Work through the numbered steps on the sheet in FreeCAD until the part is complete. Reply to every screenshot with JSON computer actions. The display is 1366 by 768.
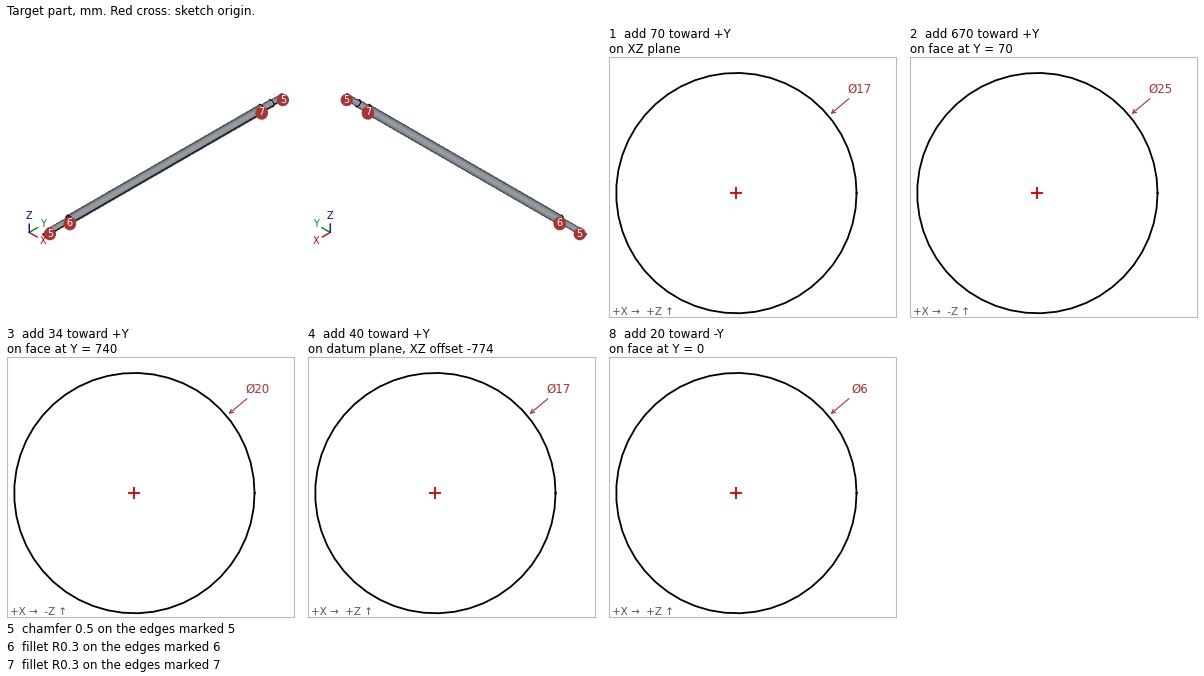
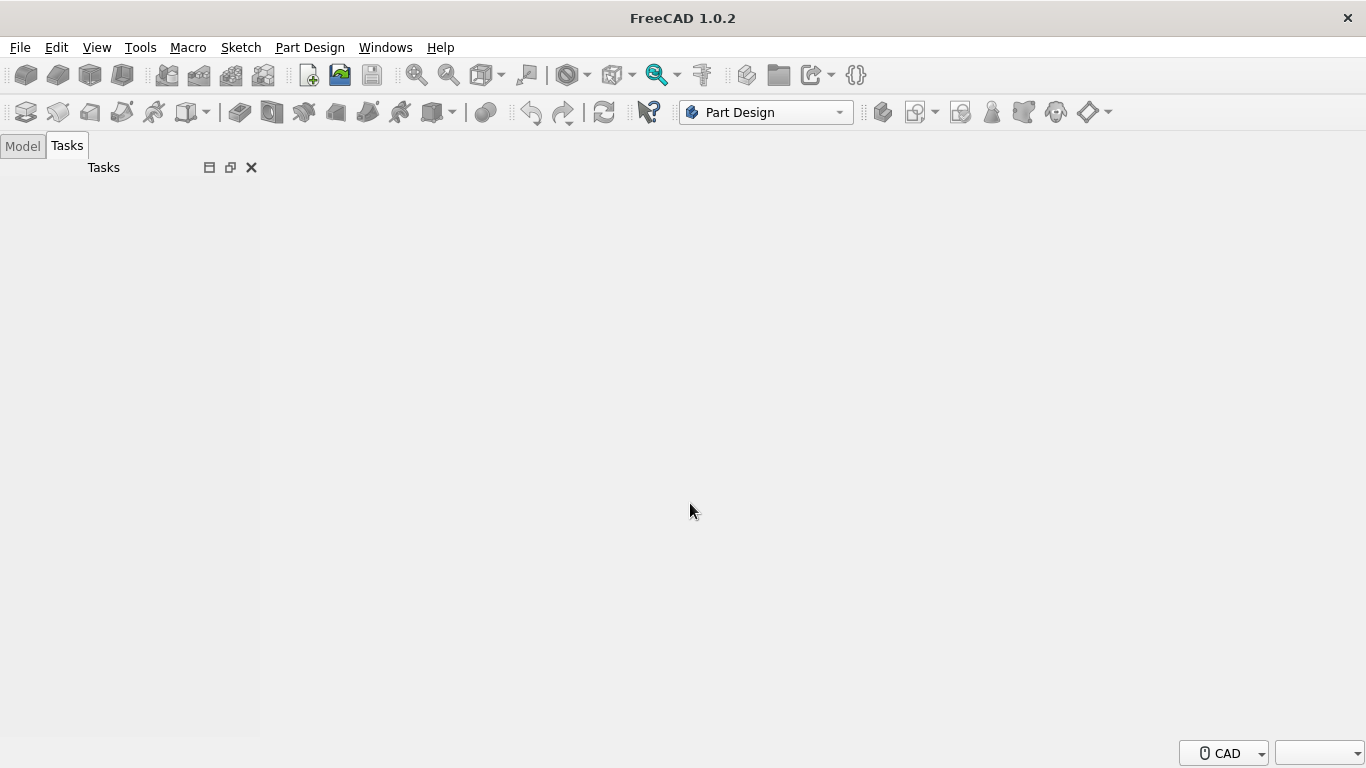
{"action": "left_click", "coordinate": [308, 76]}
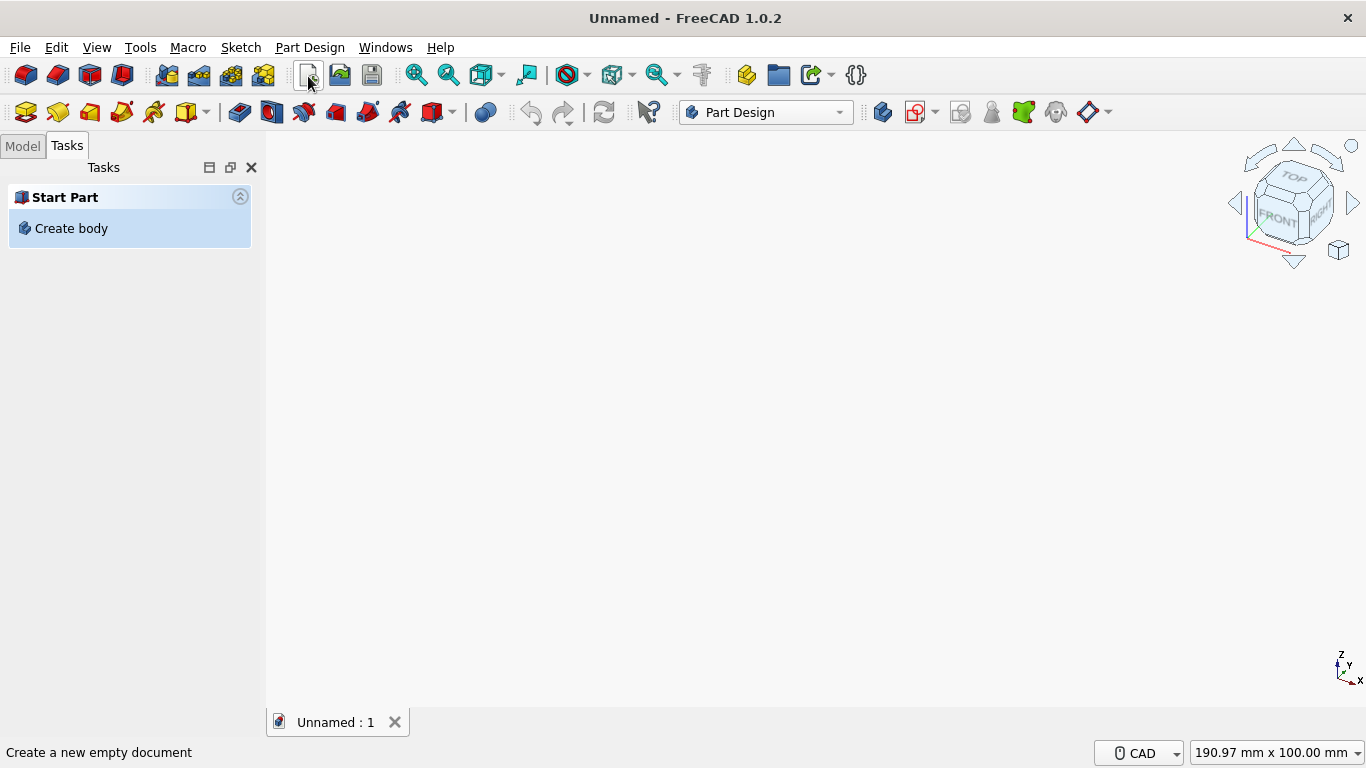
{"action": "left_click", "coordinate": [916, 112]}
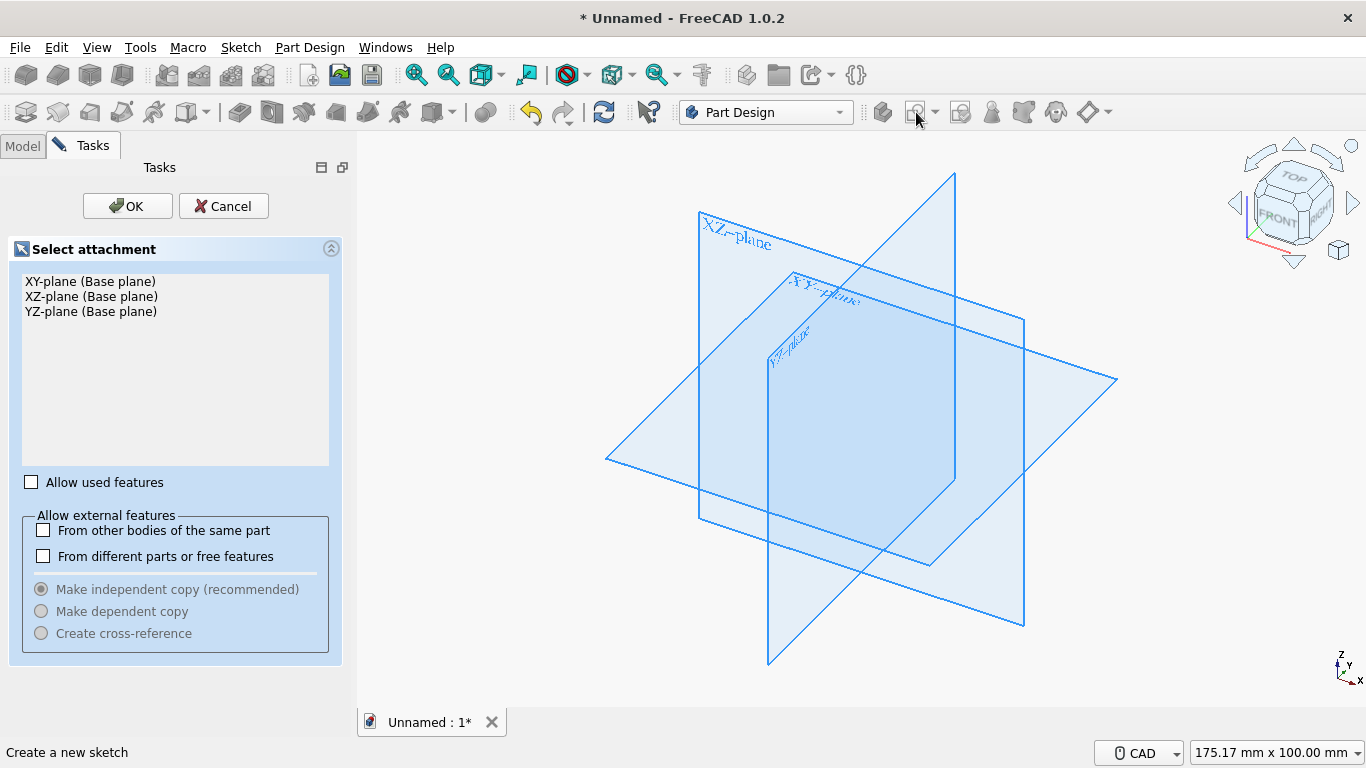
{"action": "left_click", "coordinate": [82, 296]}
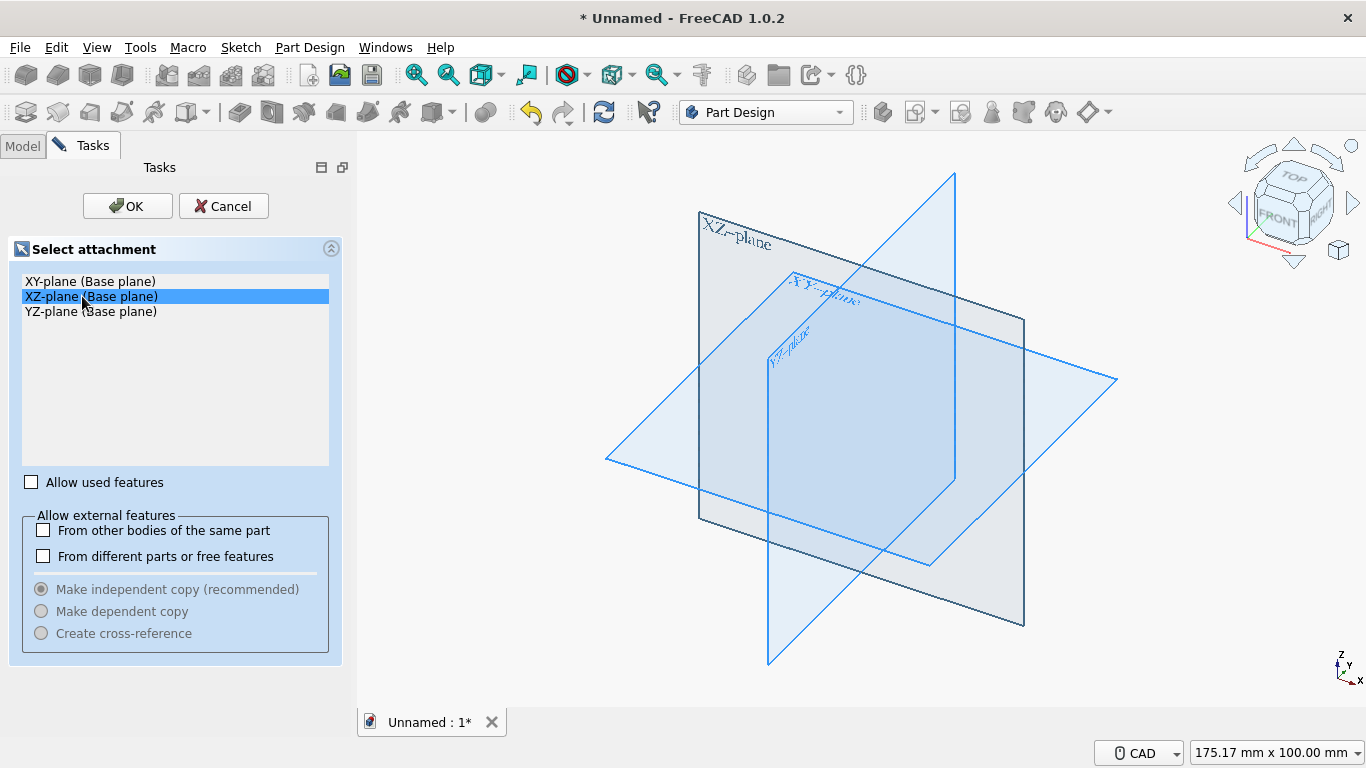
{"action": "left_click", "coordinate": [128, 206]}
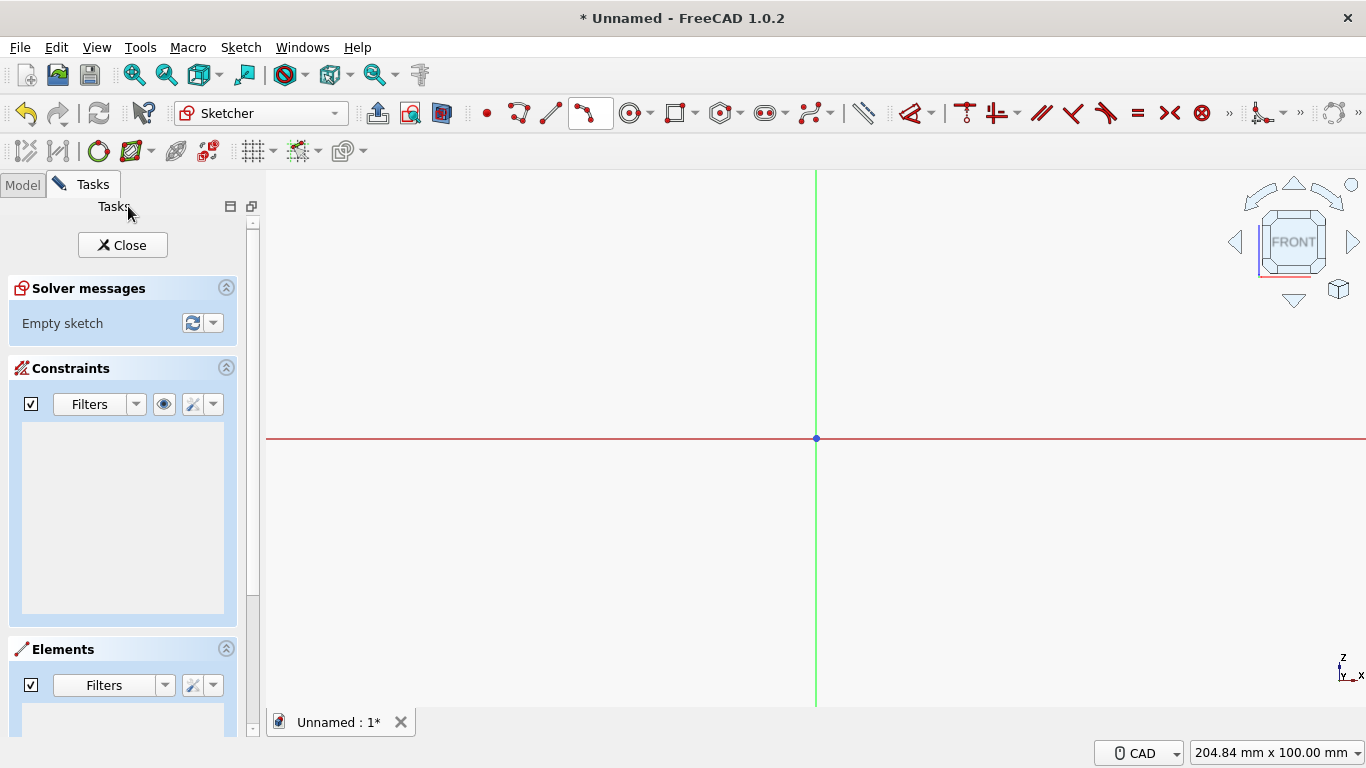
{"action": "scroll", "coordinate": [838, 438], "scroll_direction": "up", "scroll_amount": 7}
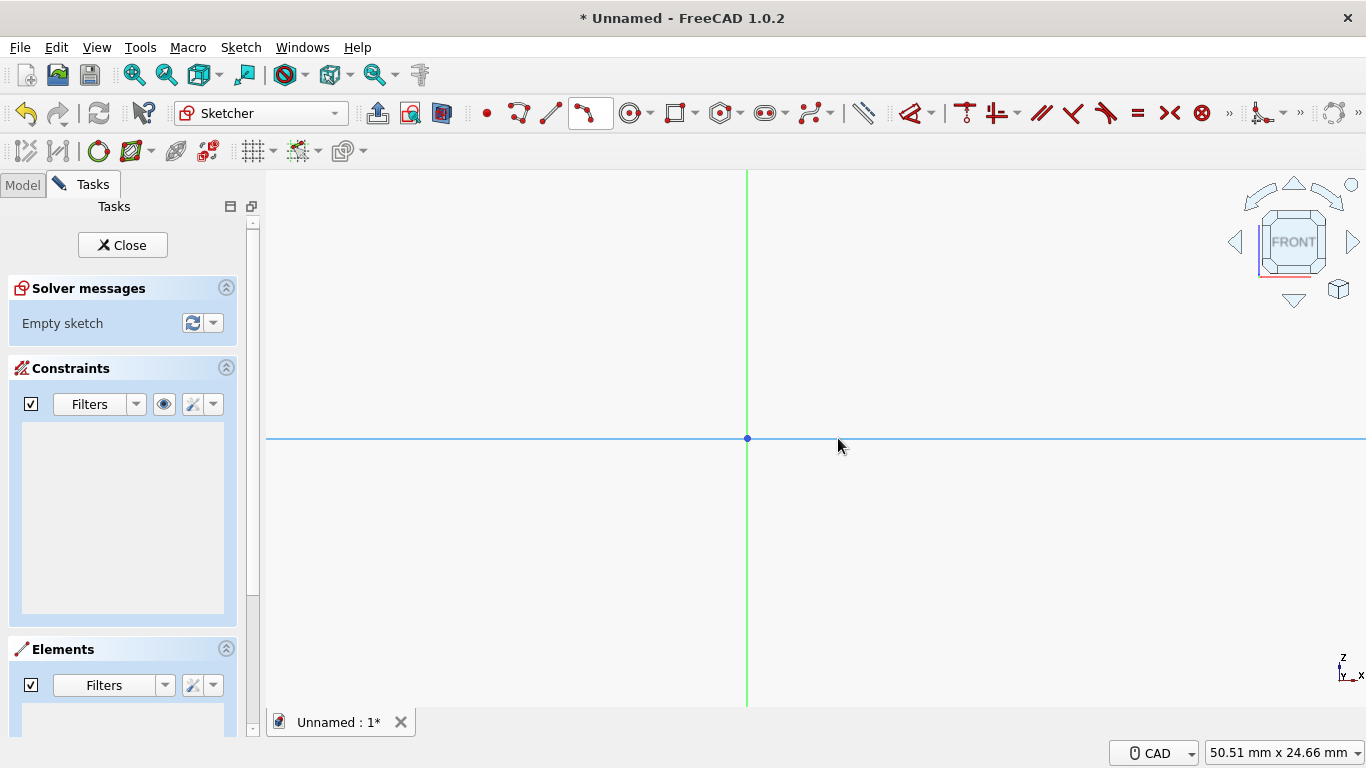
{"action": "left_click", "coordinate": [630, 114]}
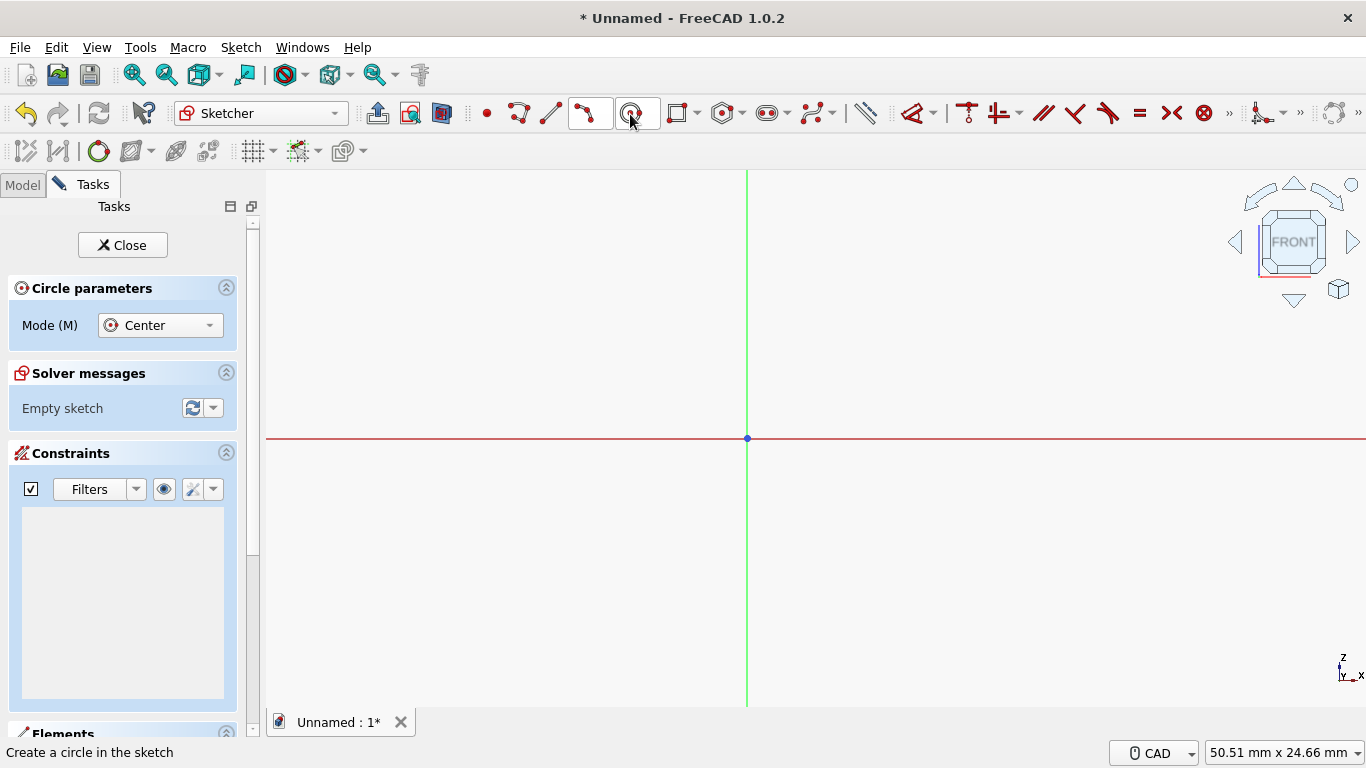
{"action": "left_click", "coordinate": [747, 438]}
{"action": "left_click", "coordinate": [878, 308]}
{"action": "key", "text": "Escape"}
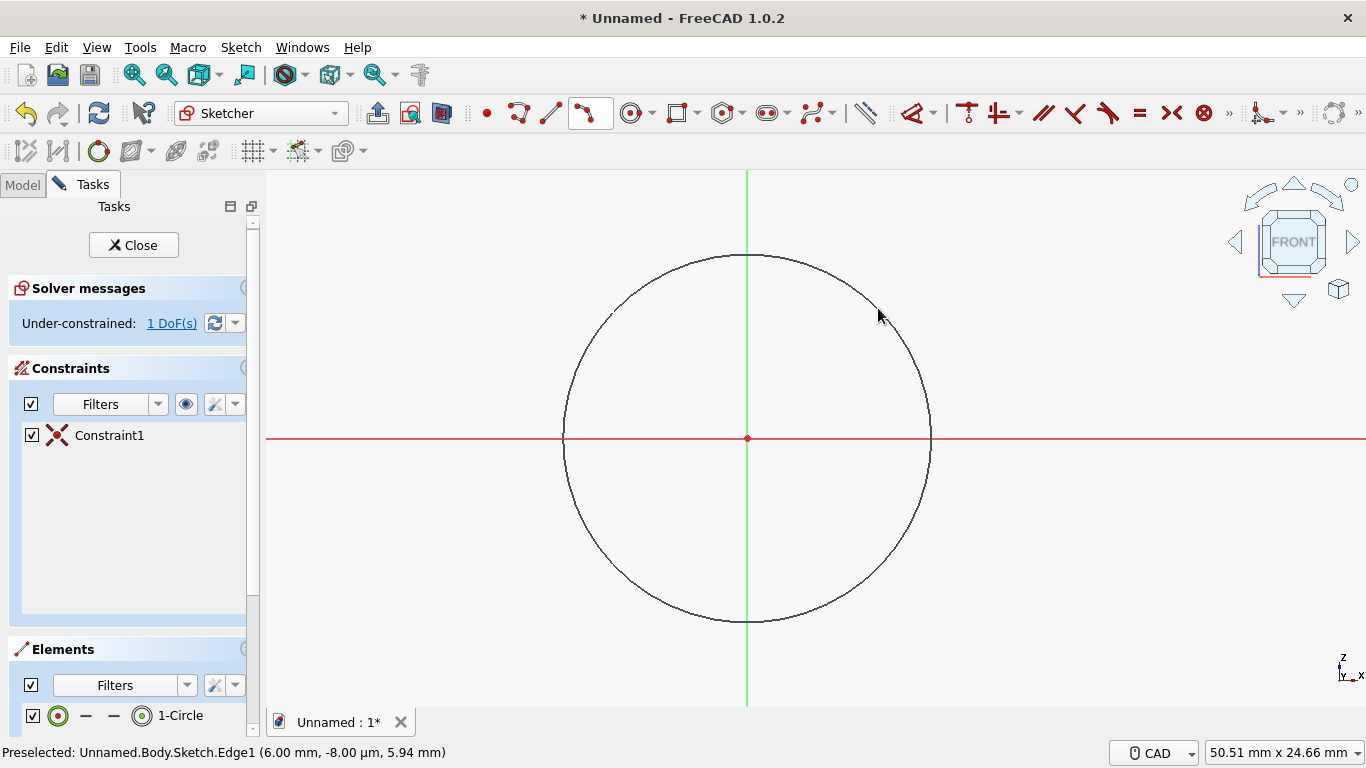
{"action": "left_click", "coordinate": [912, 114]}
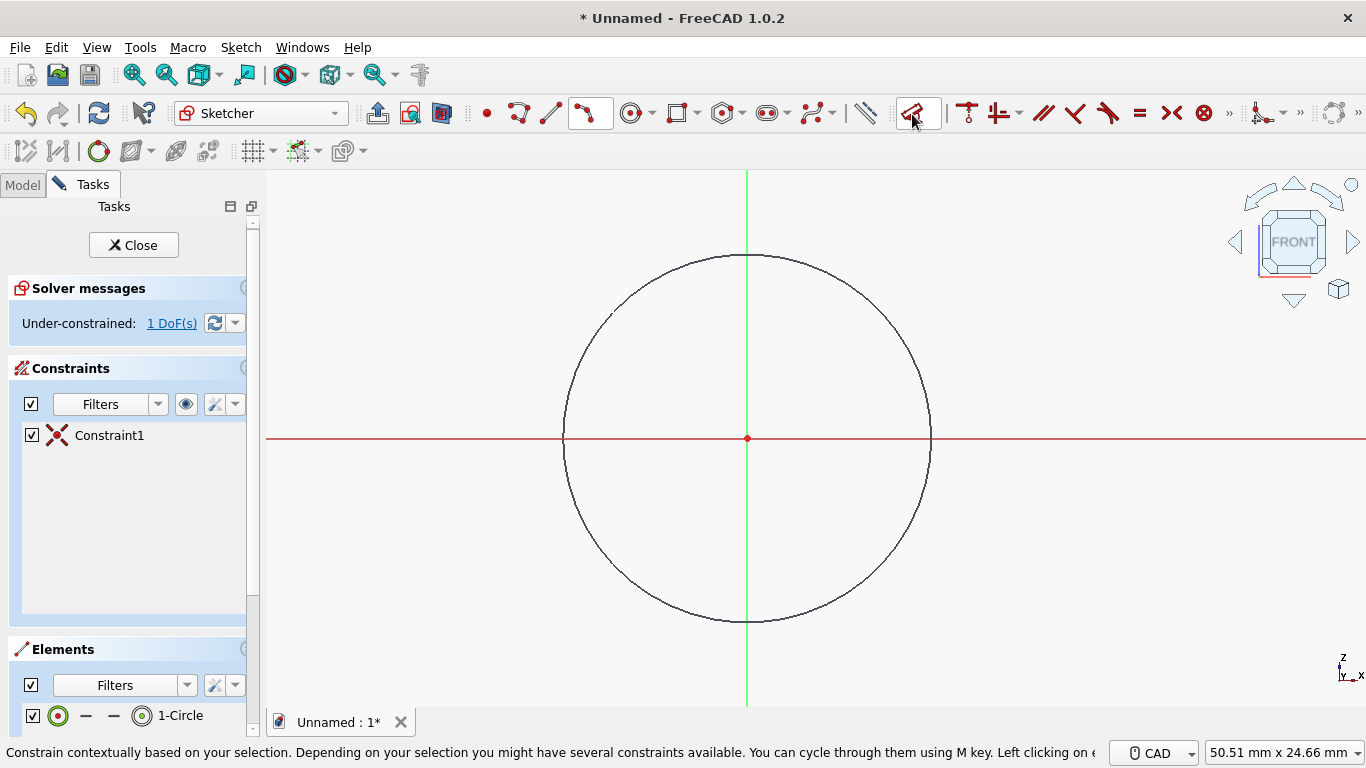
{"action": "left_click", "coordinate": [877, 308]}
{"action": "left_click", "coordinate": [900, 285]}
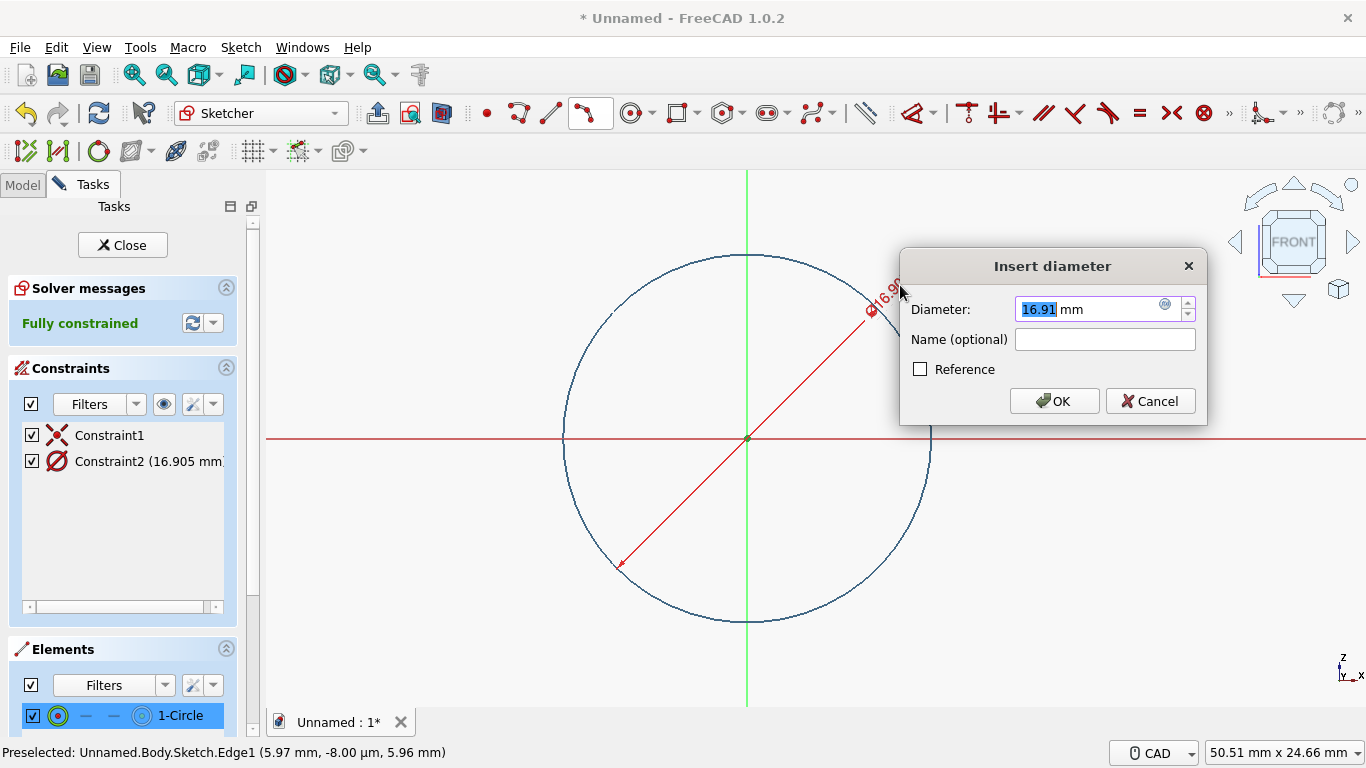
{"action": "type", "text": "17"}
{"action": "key", "text": "Return"}
{"action": "key", "text": "Escape"}